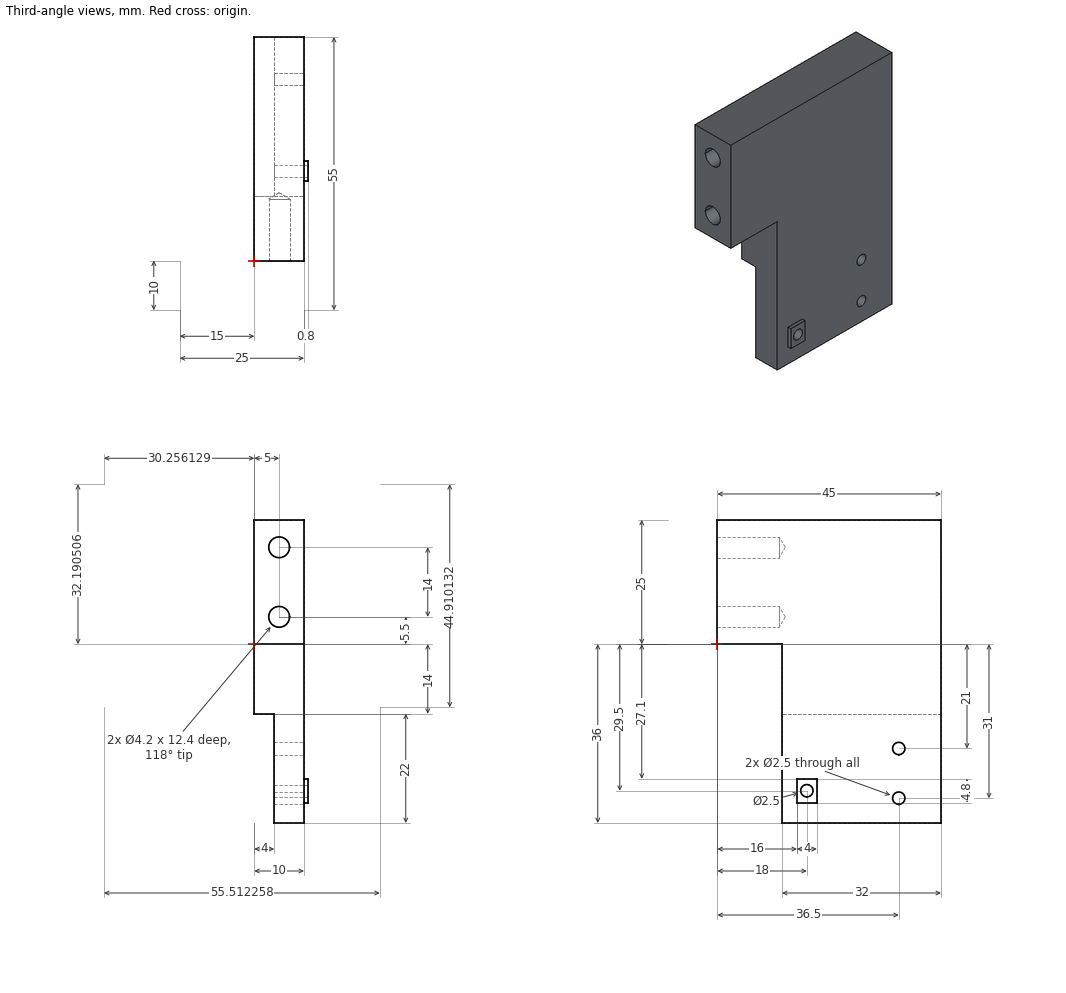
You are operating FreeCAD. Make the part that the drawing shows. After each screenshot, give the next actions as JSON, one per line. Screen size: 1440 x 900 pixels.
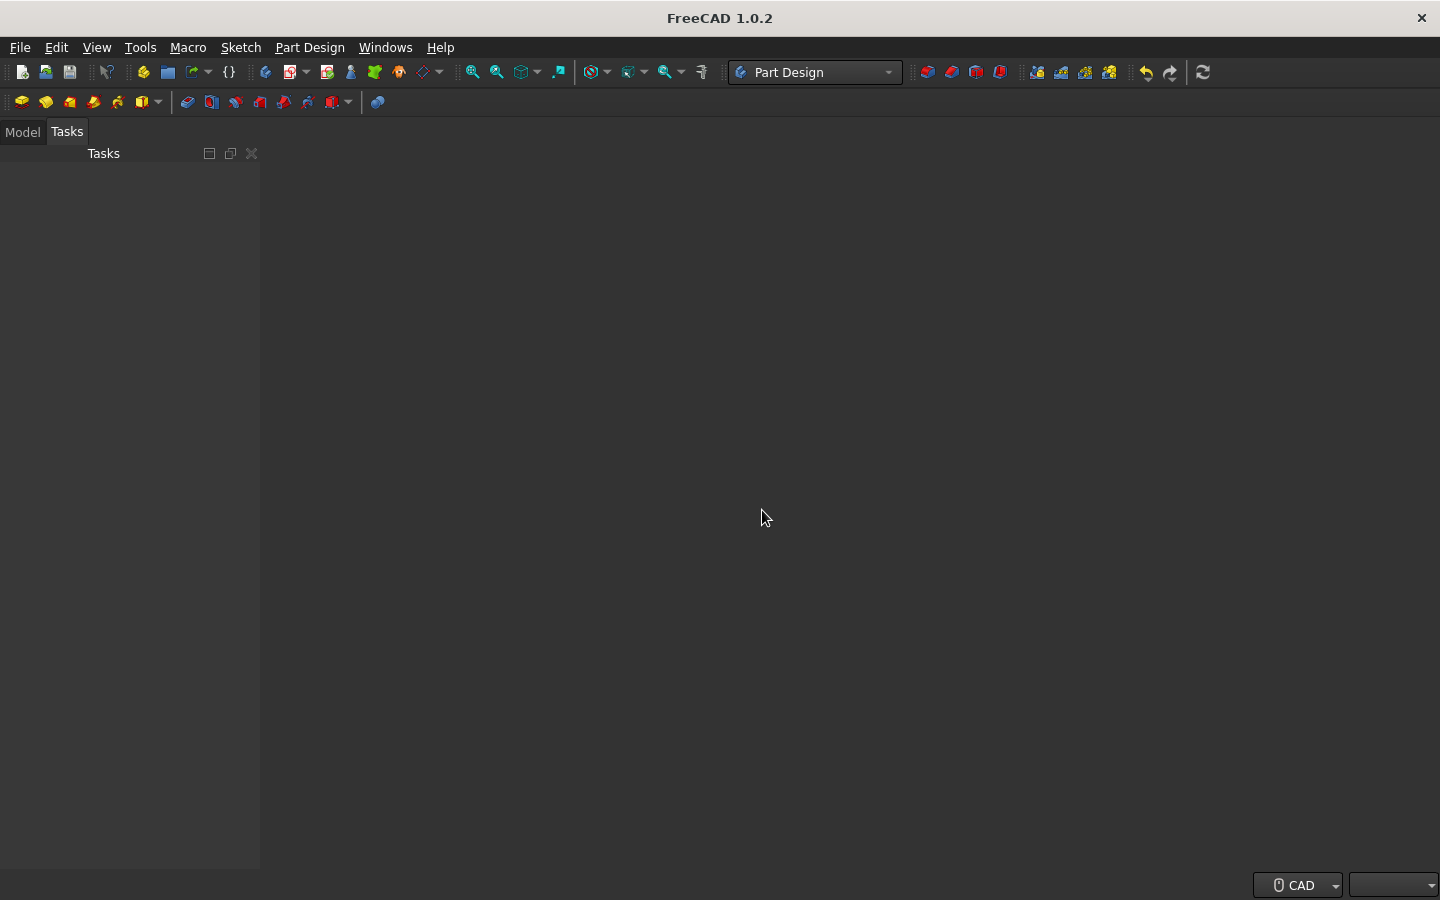
{"action": "left_click", "coordinate": [22, 72]}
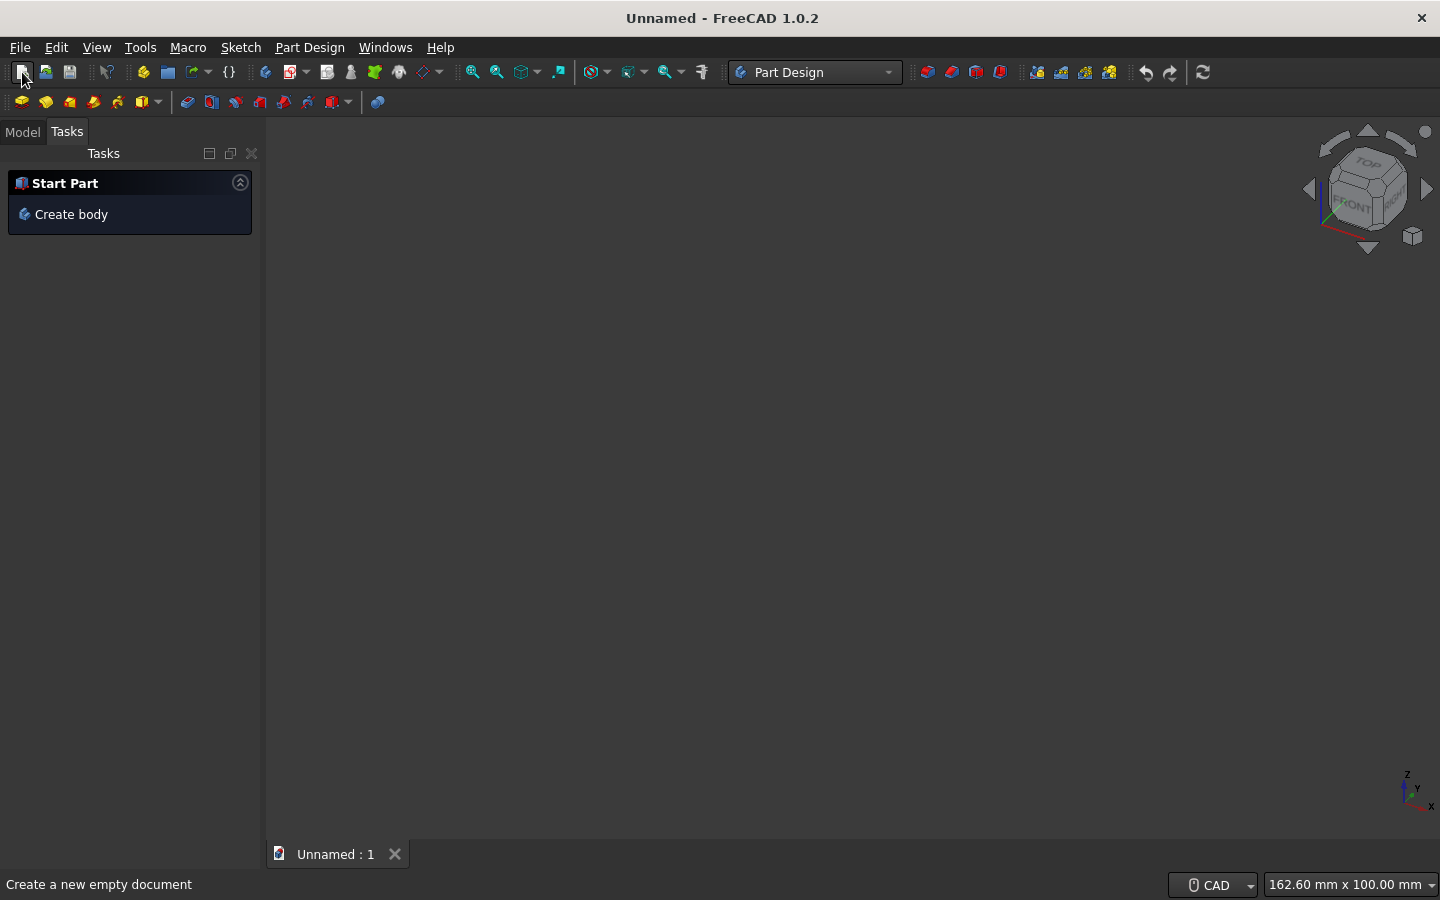
{"action": "left_click", "coordinate": [290, 72]}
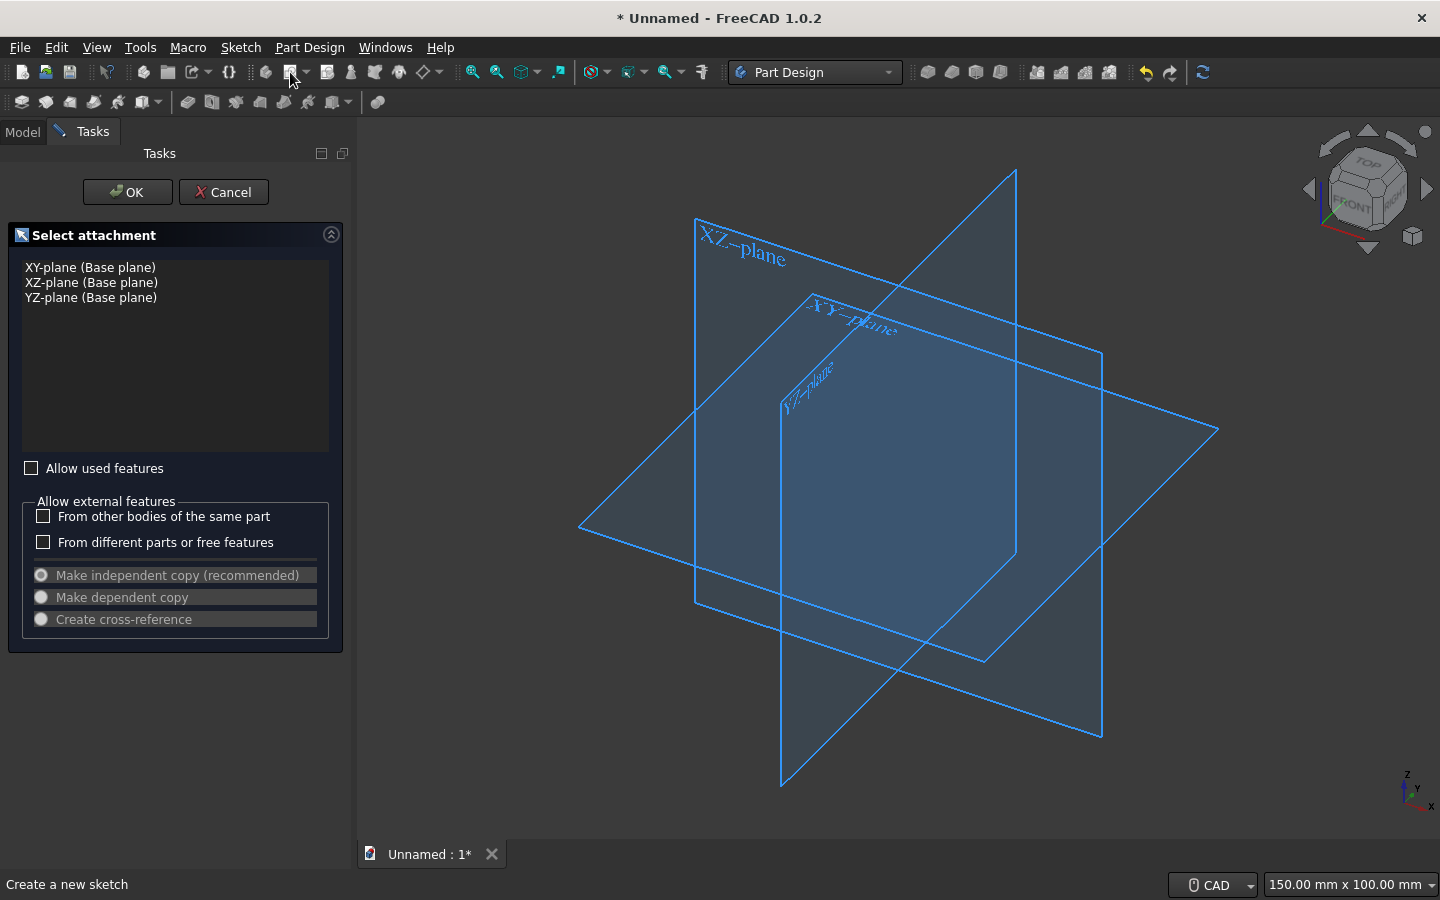
{"action": "left_click", "coordinate": [82, 268]}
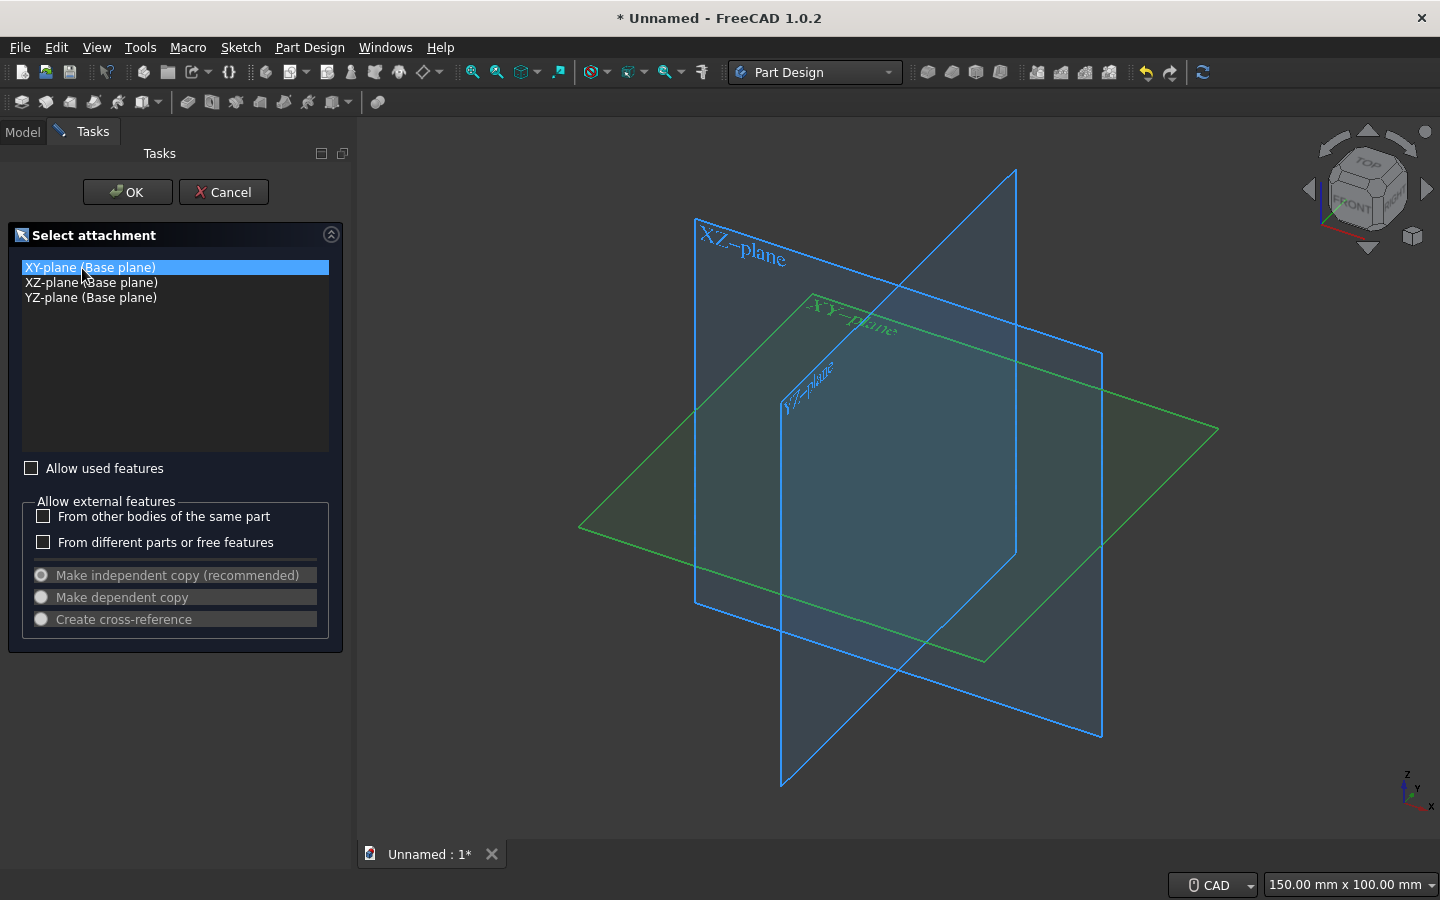
{"action": "left_click", "coordinate": [128, 192]}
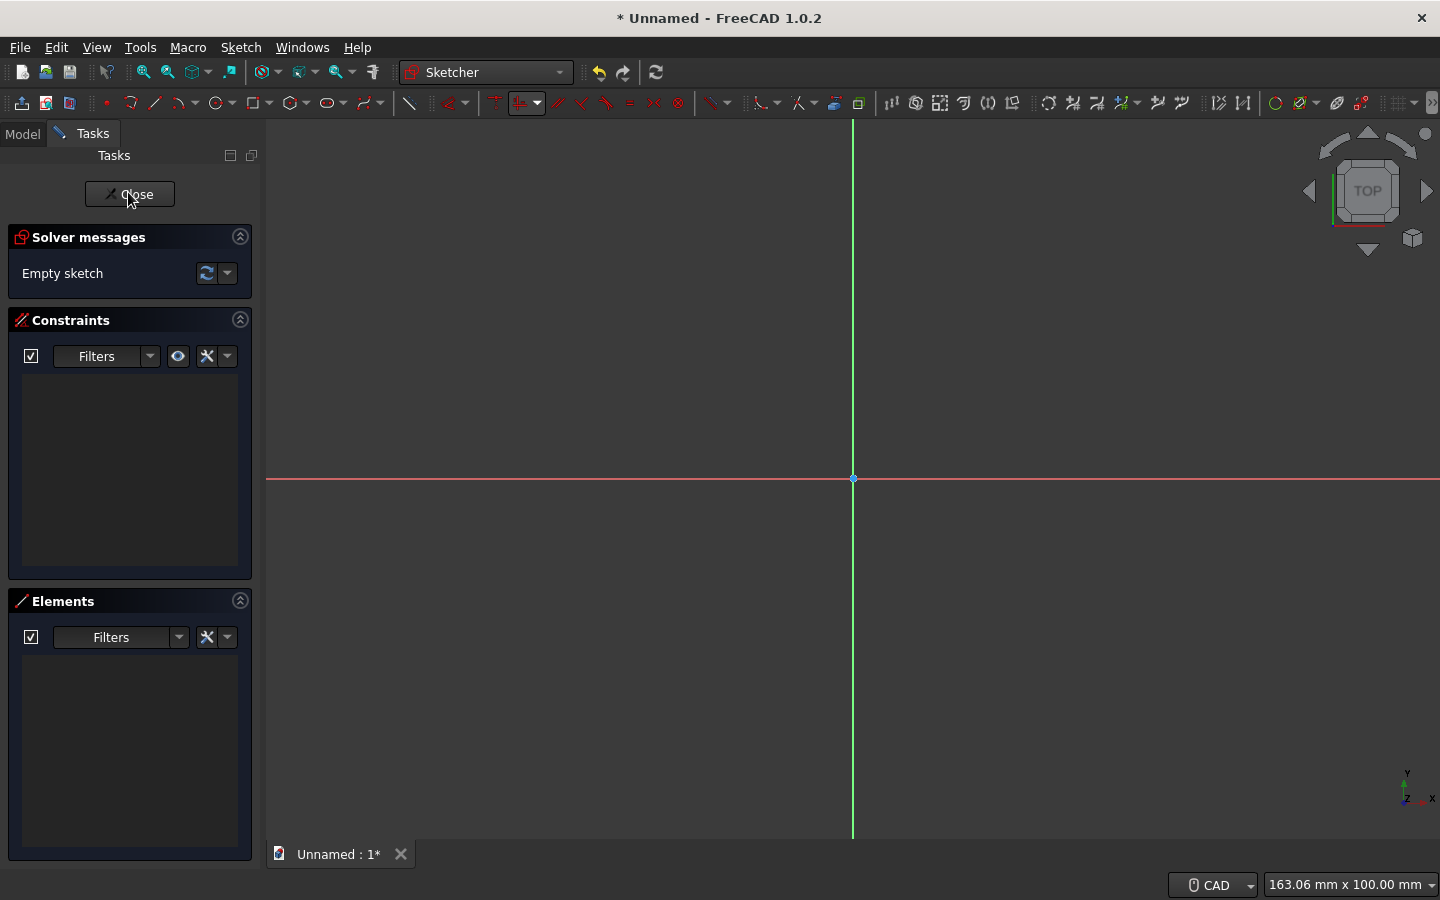
{"action": "scroll", "coordinate": [556, 811], "scroll_direction": "down", "scroll_amount": 1}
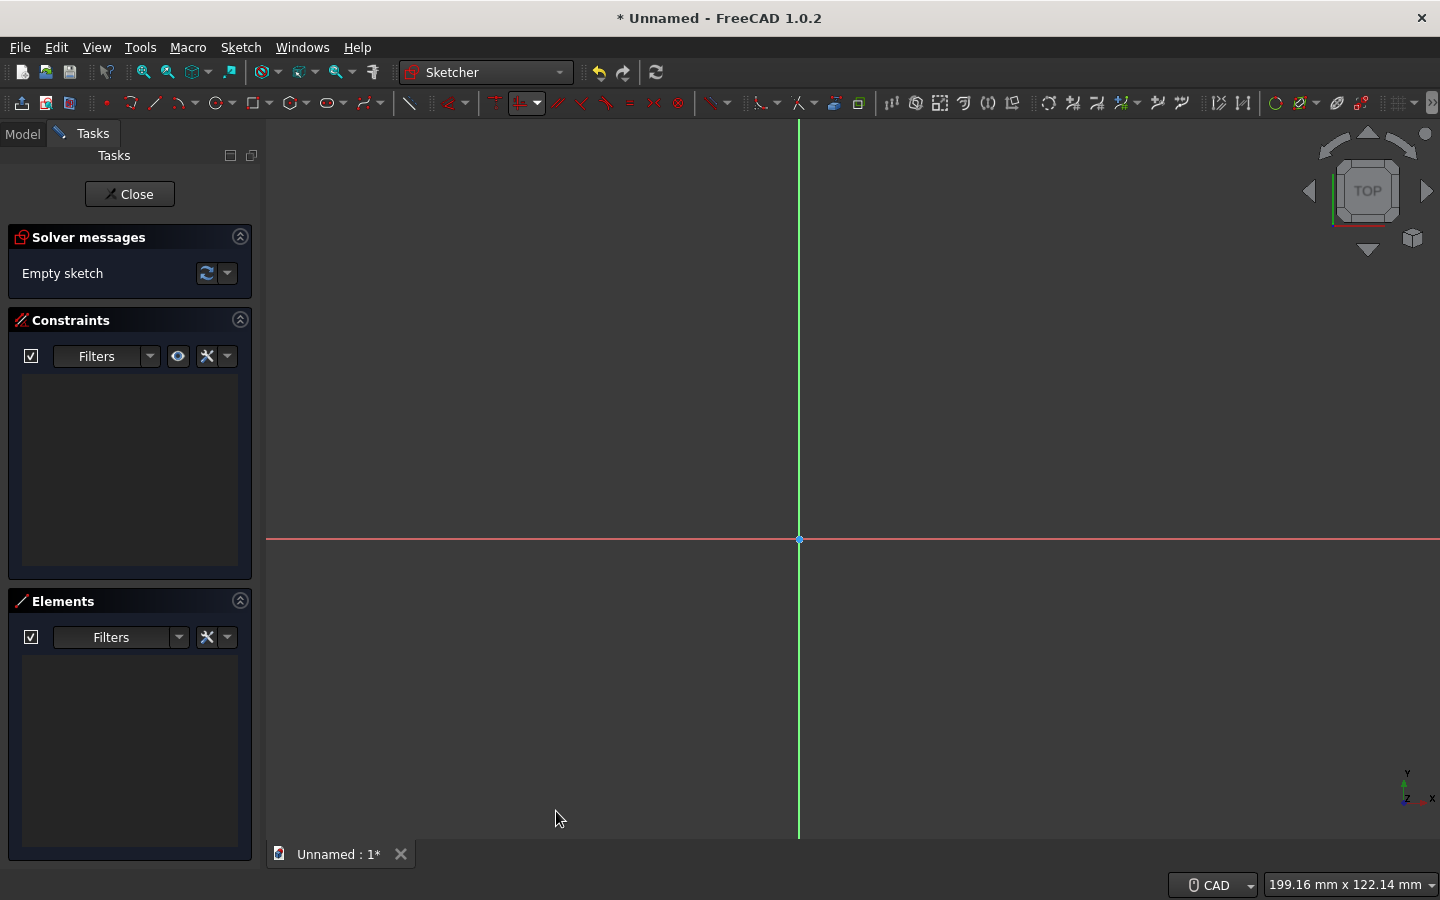
{"action": "scroll", "coordinate": [784, 349], "scroll_direction": "up", "scroll_amount": 2}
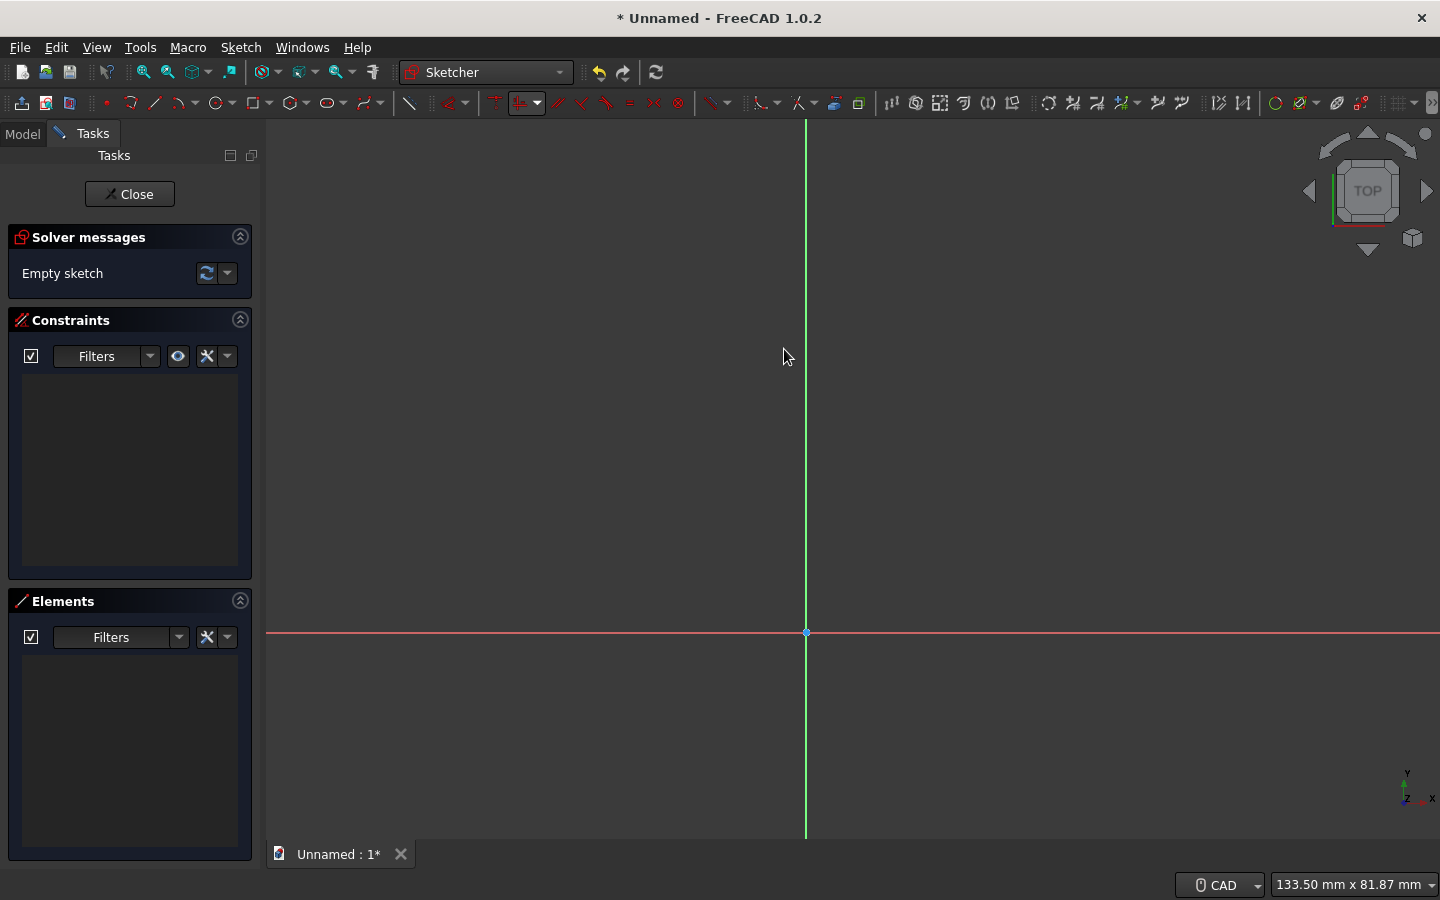
{"action": "key", "text": "g m"}